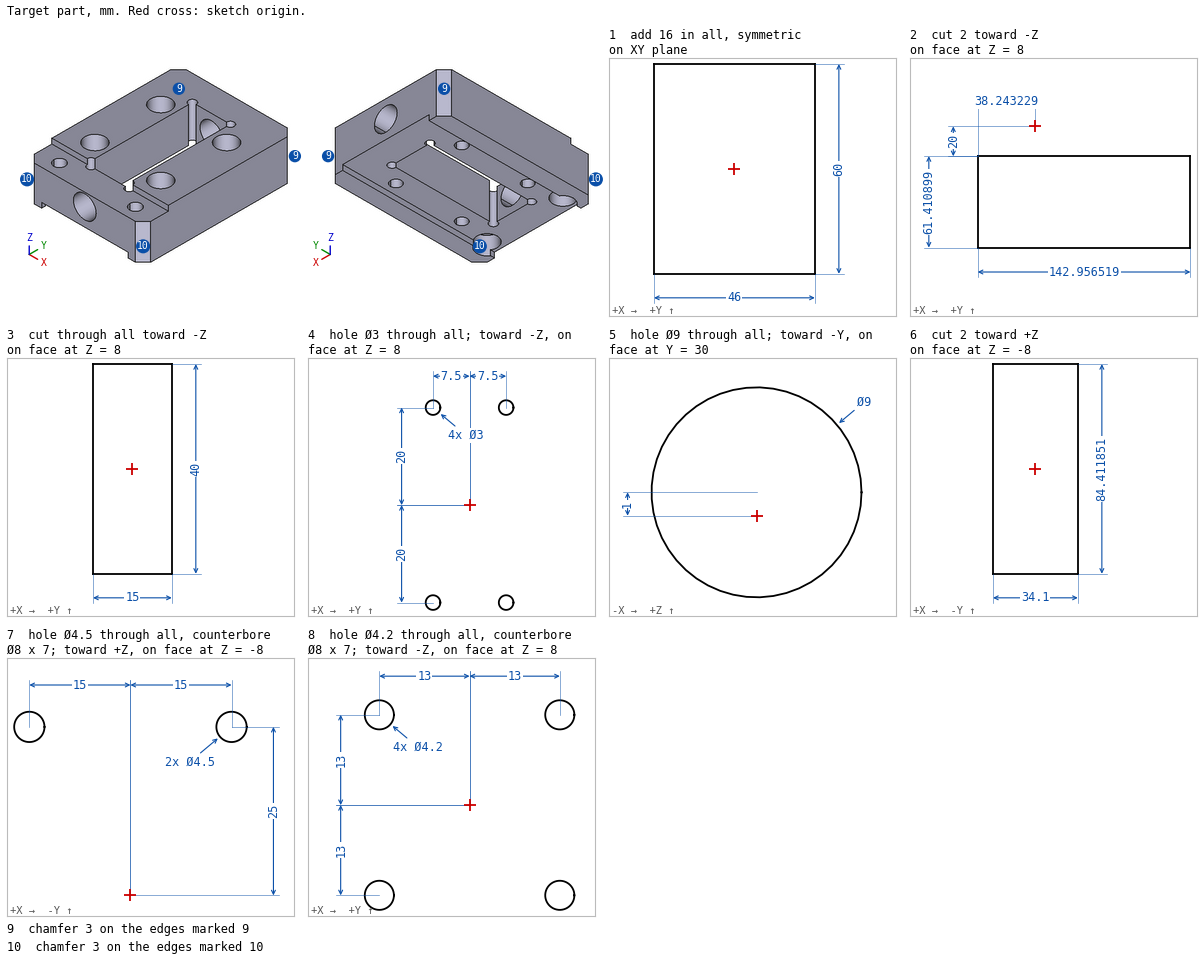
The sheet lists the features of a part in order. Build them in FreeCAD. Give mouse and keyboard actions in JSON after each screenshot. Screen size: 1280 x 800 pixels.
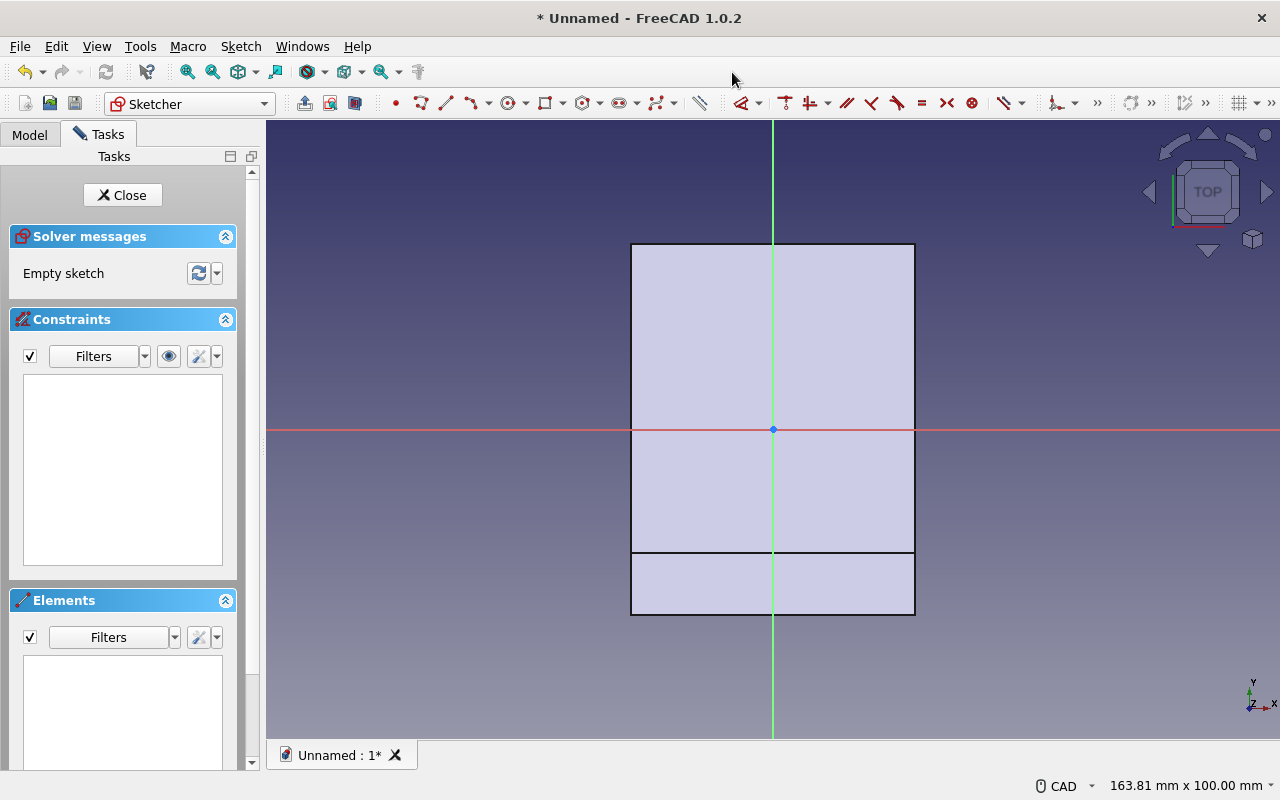
{"action": "scroll", "coordinate": [912, 429], "scroll_direction": "up", "scroll_amount": 2}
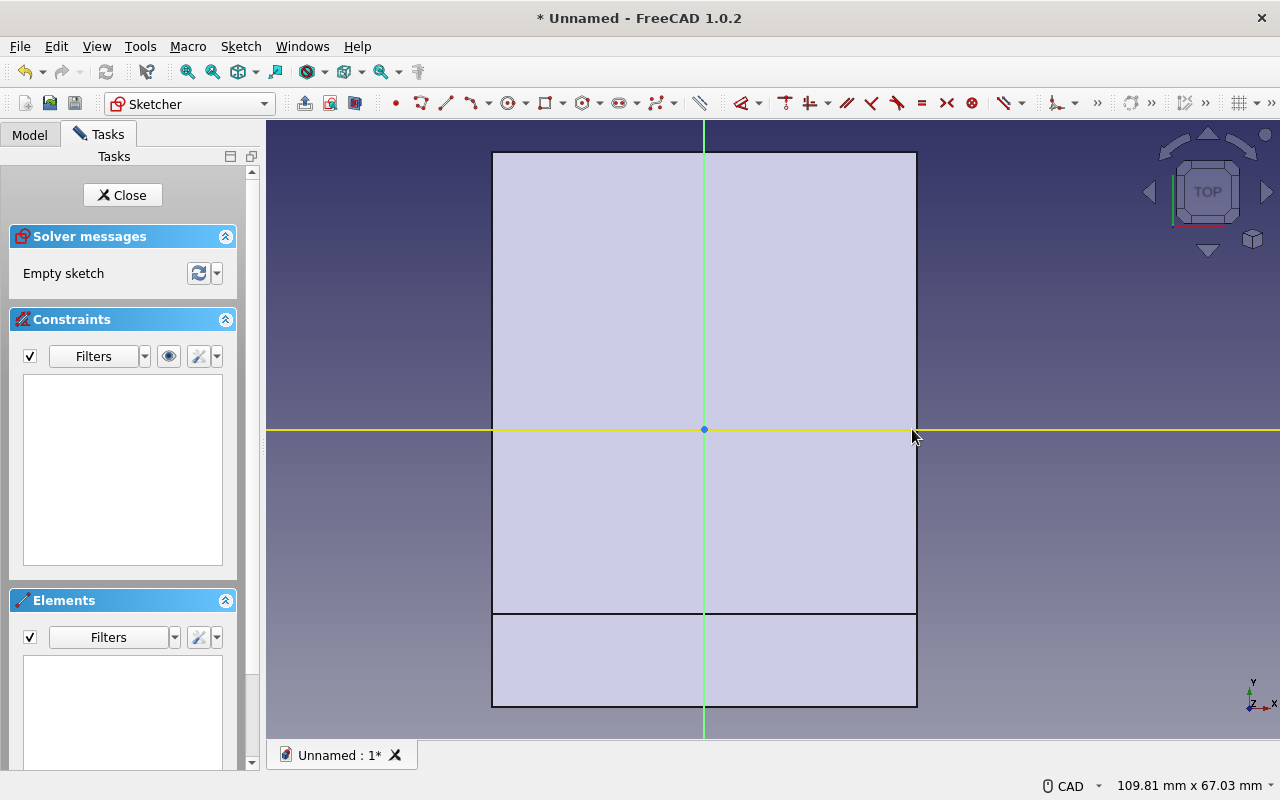
{"action": "left_click", "coordinate": [562, 104]}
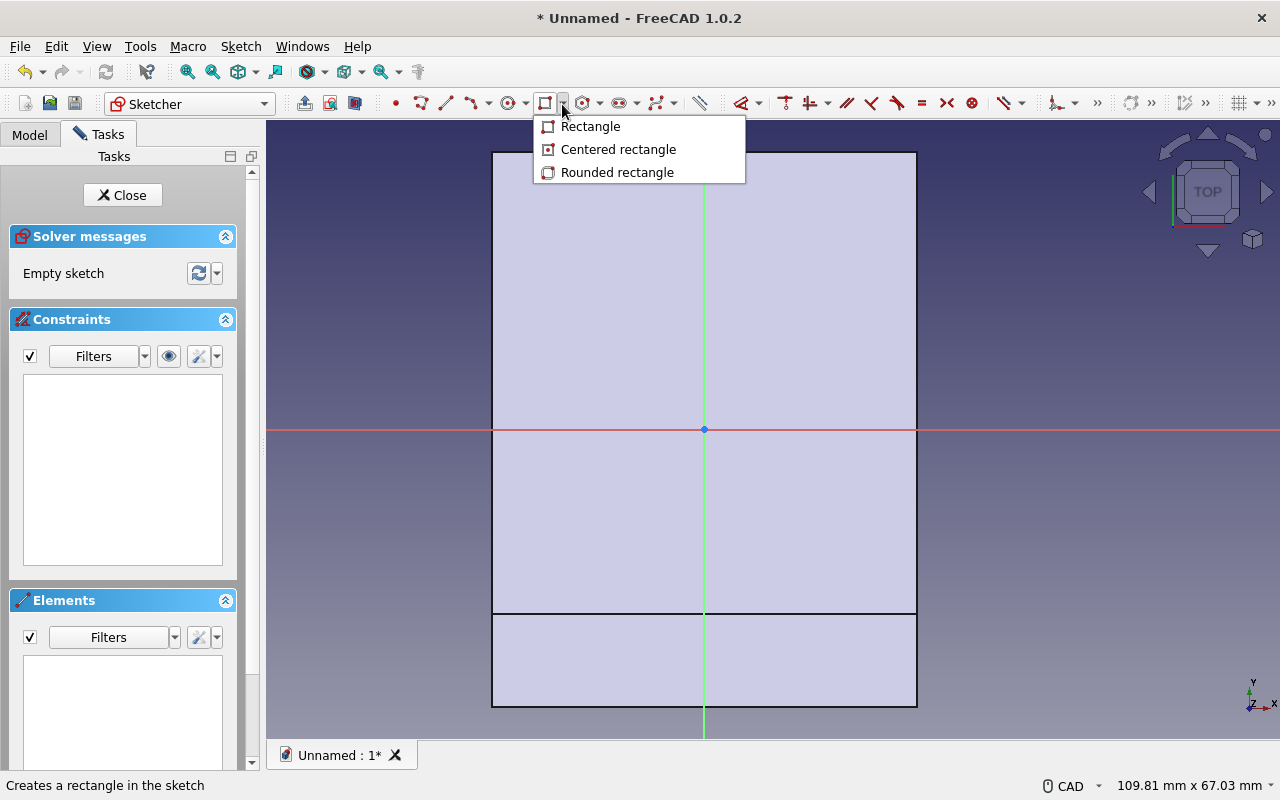
{"action": "left_click", "coordinate": [640, 150]}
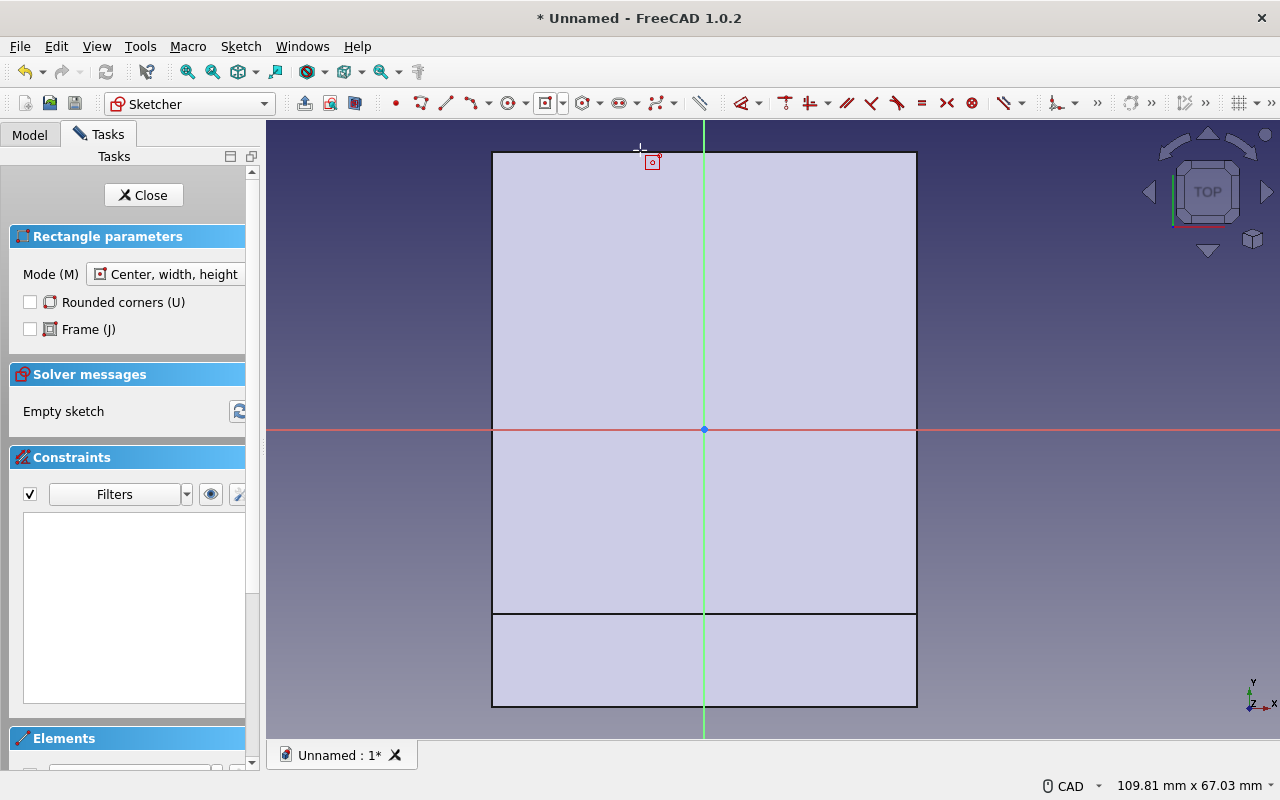
{"action": "left_click", "coordinate": [704, 430]}
{"action": "left_click", "coordinate": [774, 245]}
{"action": "key", "text": "Escape"}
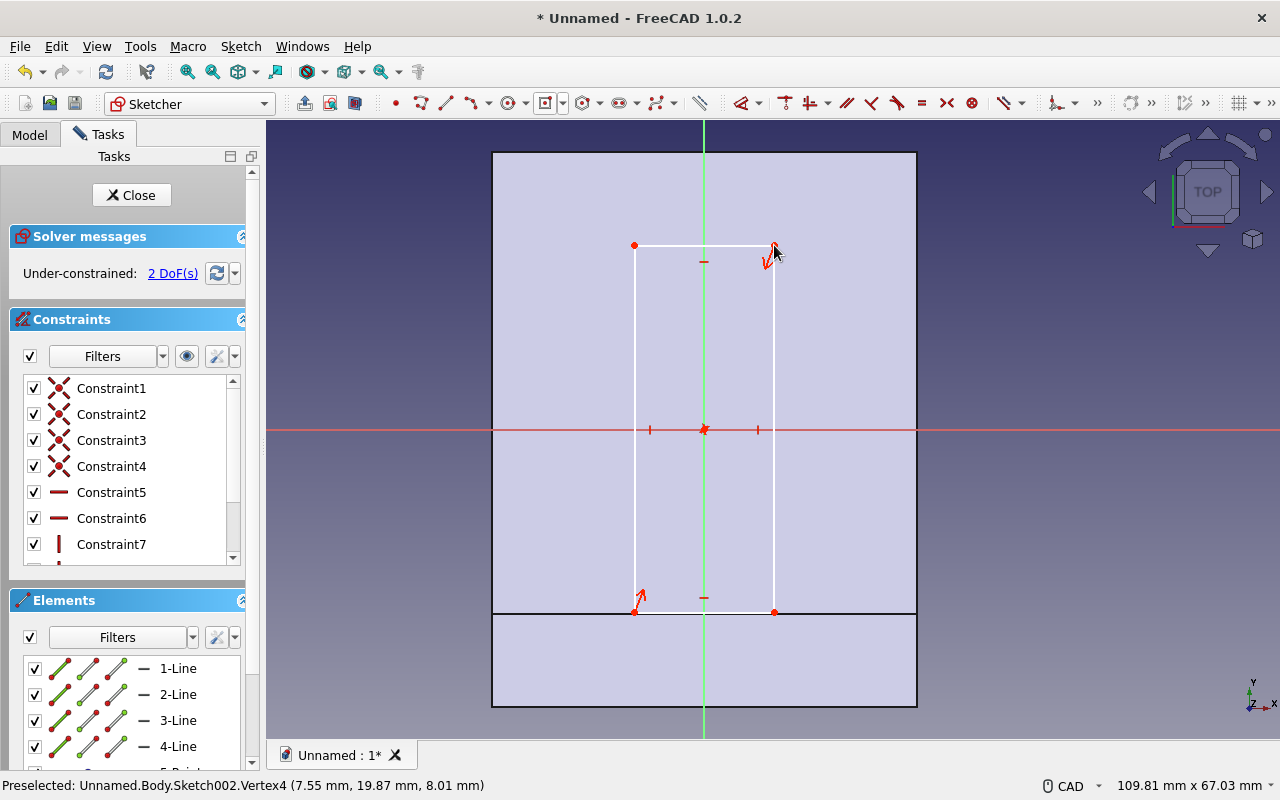
{"action": "left_click", "coordinate": [740, 104]}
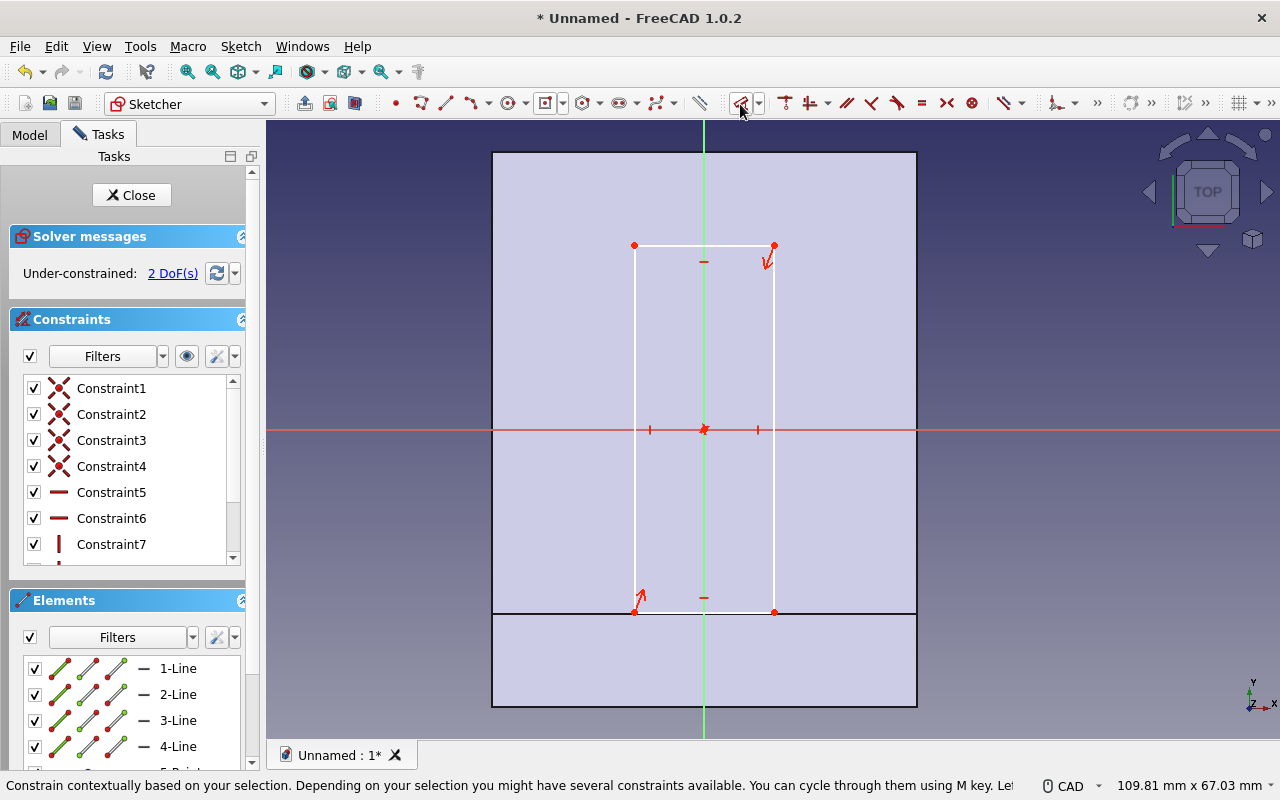
{"action": "left_click", "coordinate": [676, 613]}
{"action": "left_click", "coordinate": [672, 647]}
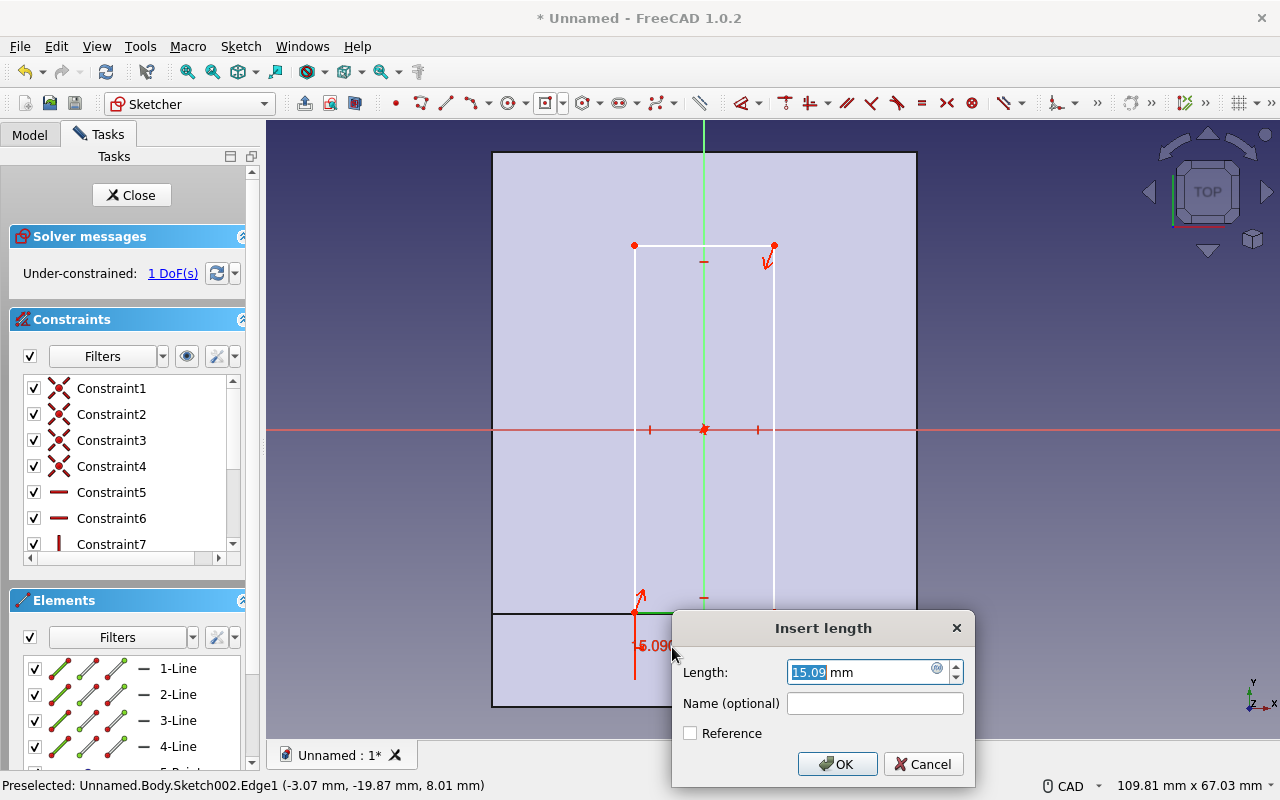
{"action": "type", "text": "15"}
{"action": "key", "text": "Return"}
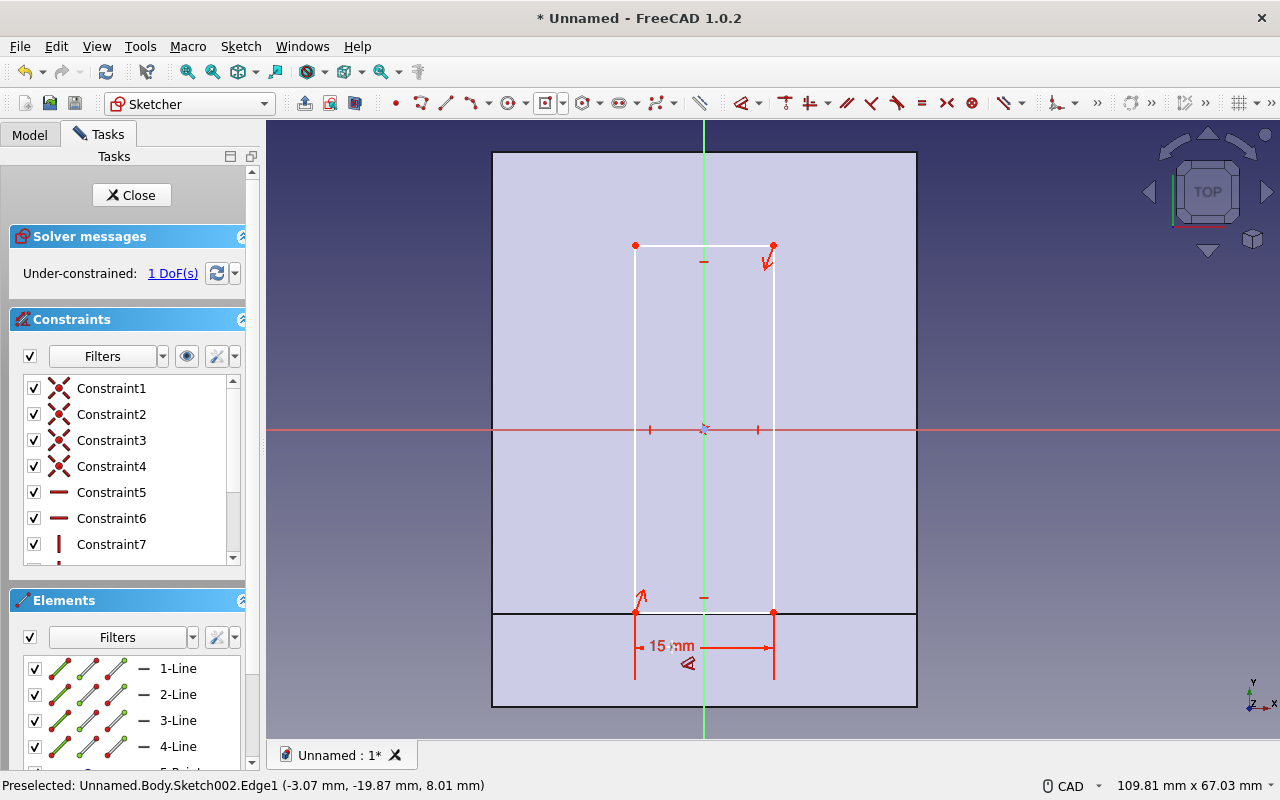
{"action": "left_click", "coordinate": [774, 503]}
{"action": "left_click", "coordinate": [808, 345]}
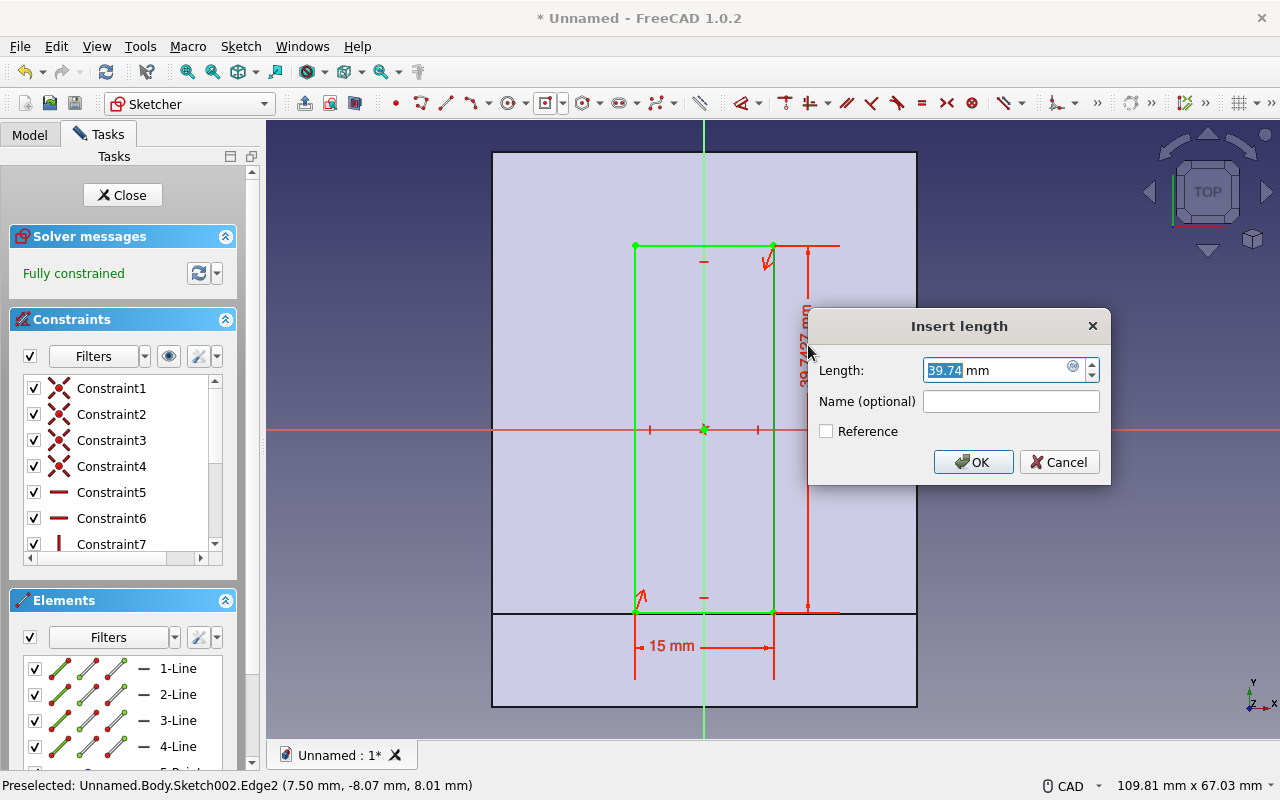
{"action": "type", "text": "40"}
{"action": "key", "text": "Return"}
{"action": "key", "text": "Escape"}